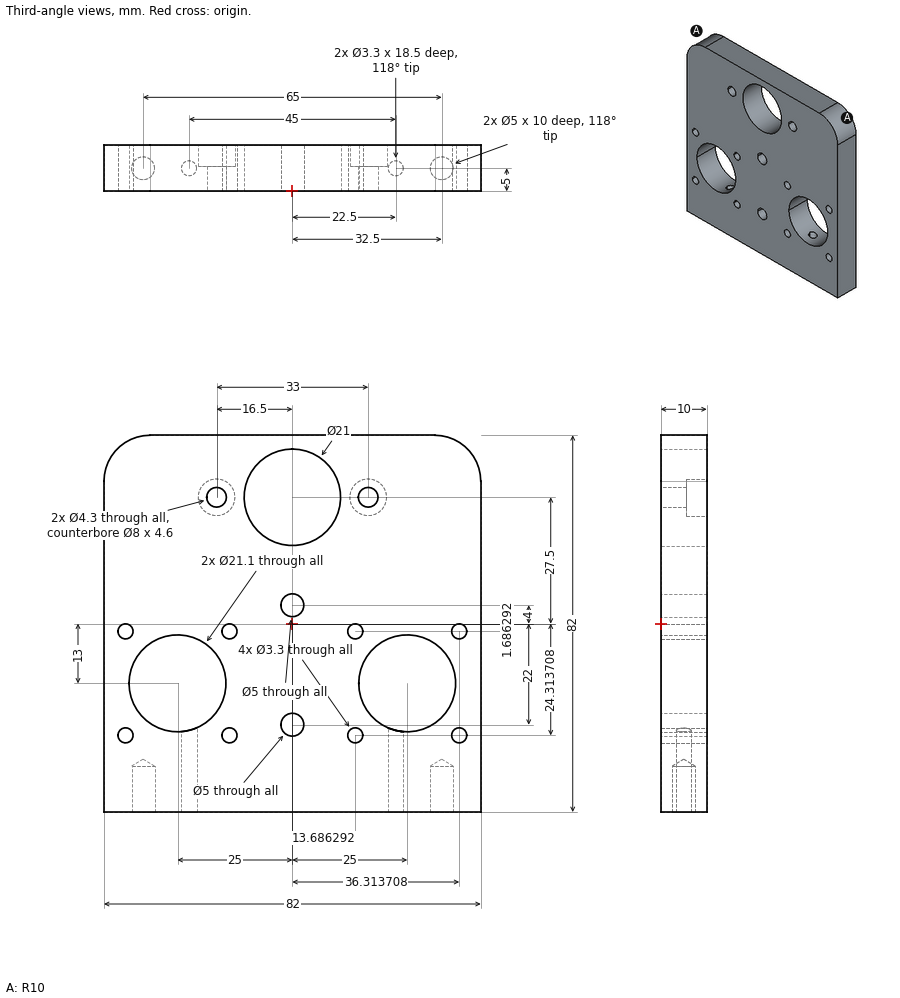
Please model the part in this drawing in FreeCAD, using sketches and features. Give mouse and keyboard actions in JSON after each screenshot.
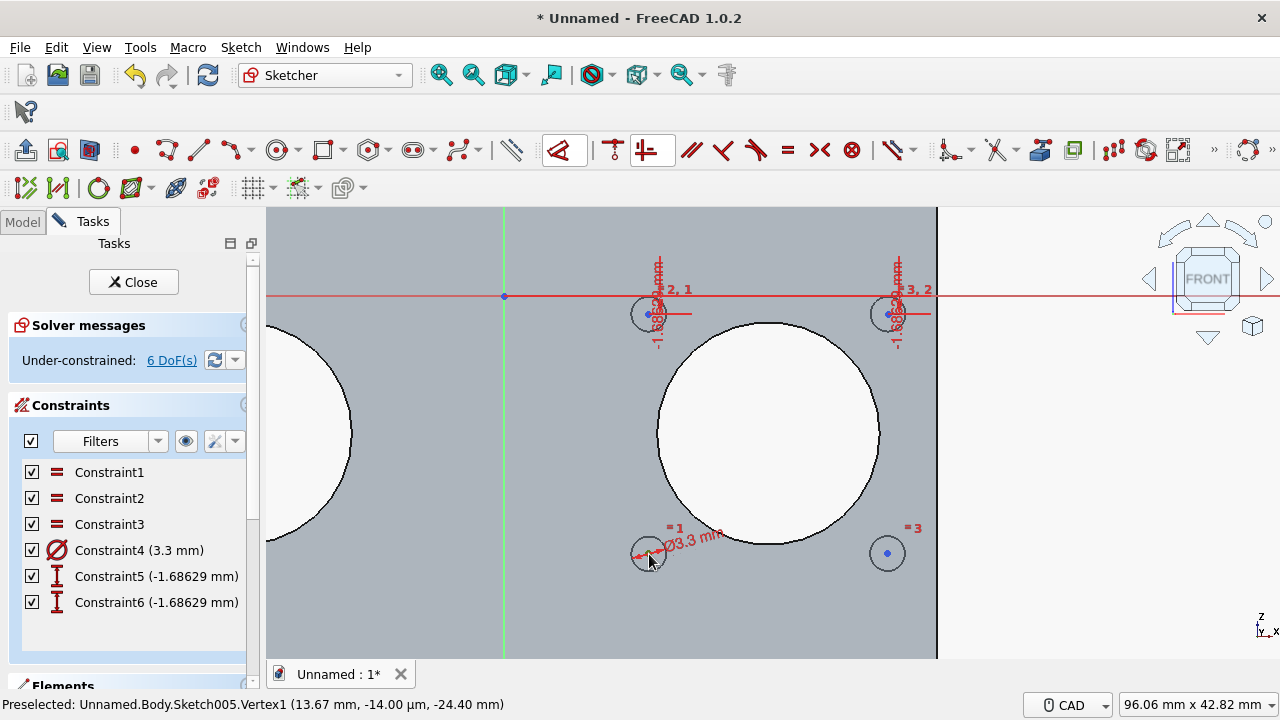
{"action": "key", "text": "l"}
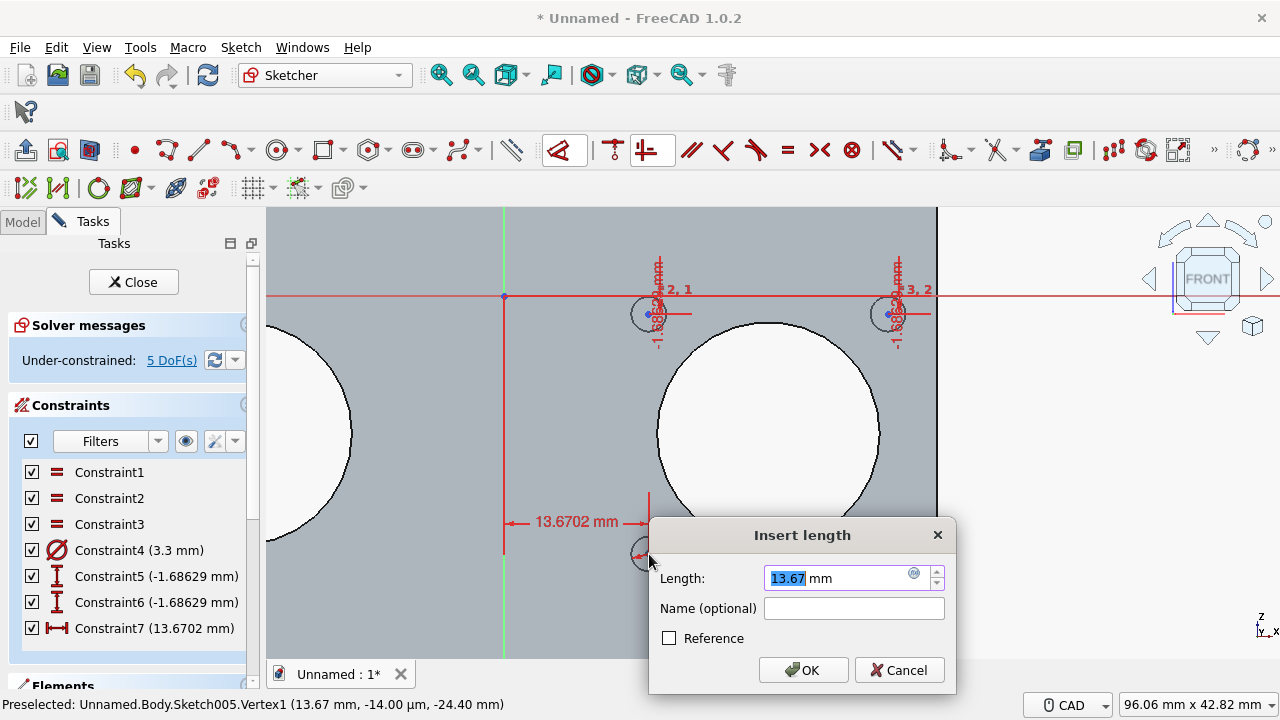
{"action": "type", "text": "13.686292"}
{"action": "key", "text": "Return"}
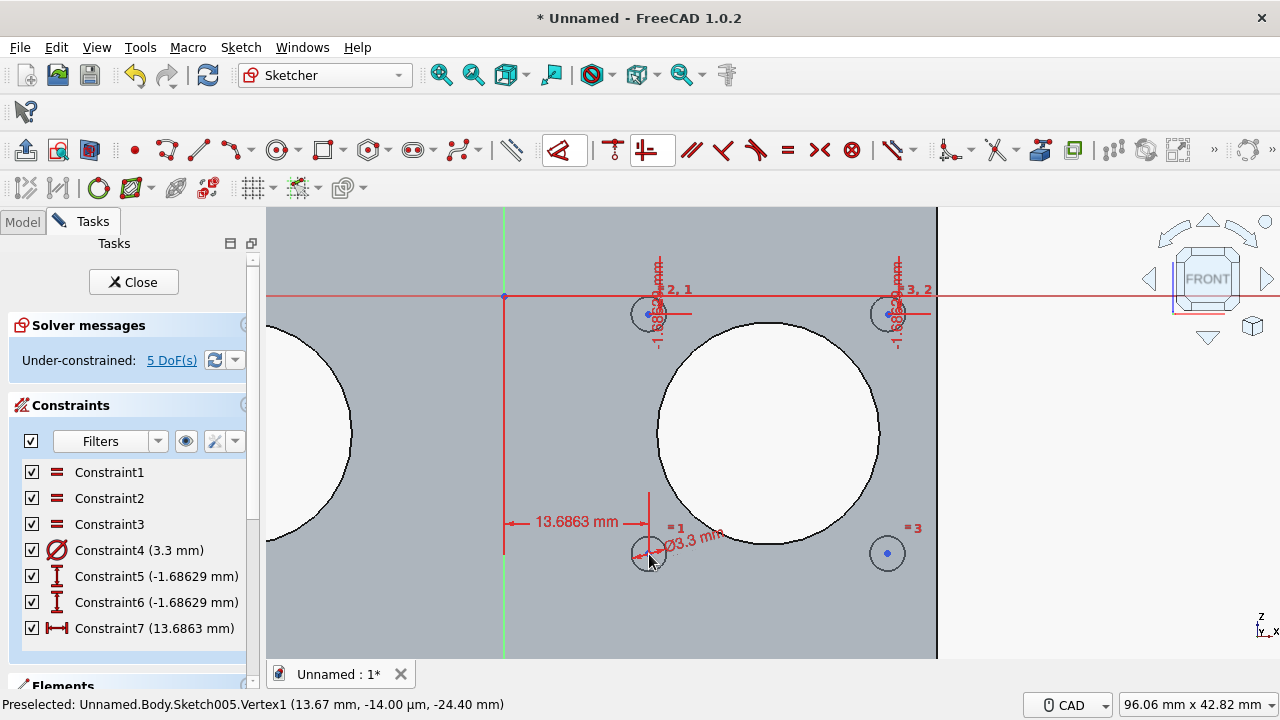
{"action": "left_click", "coordinate": [649, 554]}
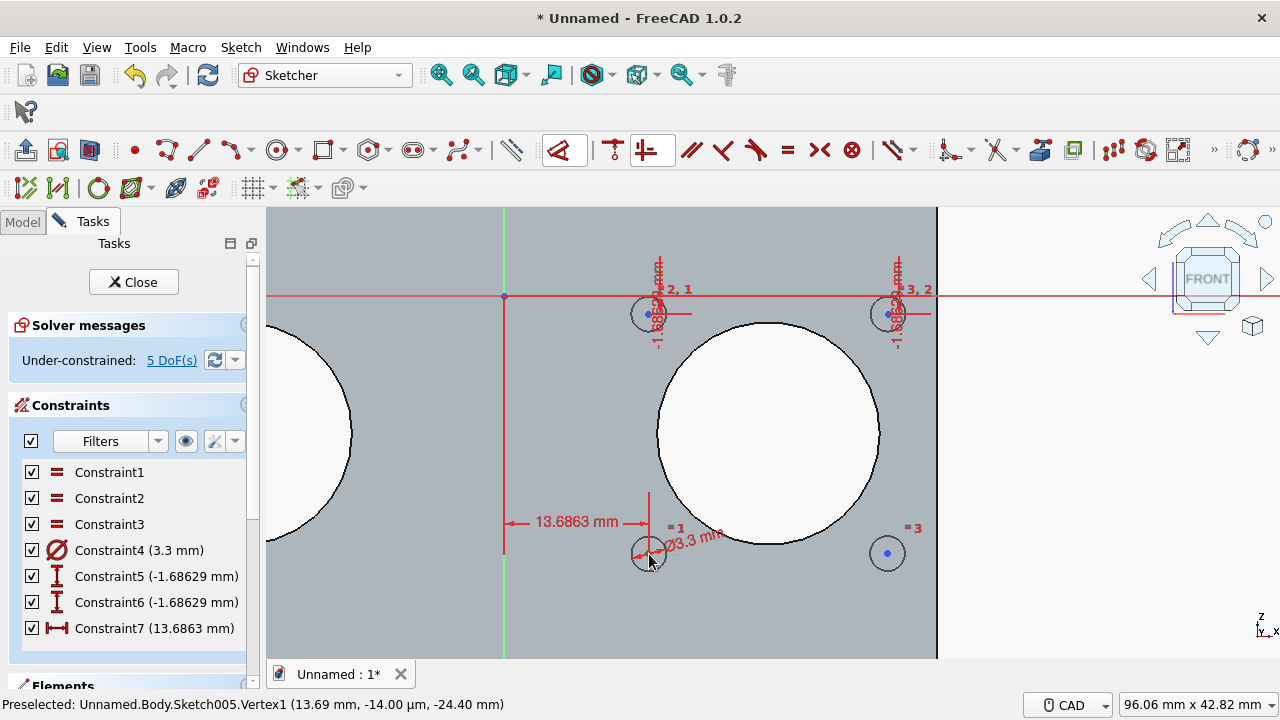
{"action": "key", "text": "i"}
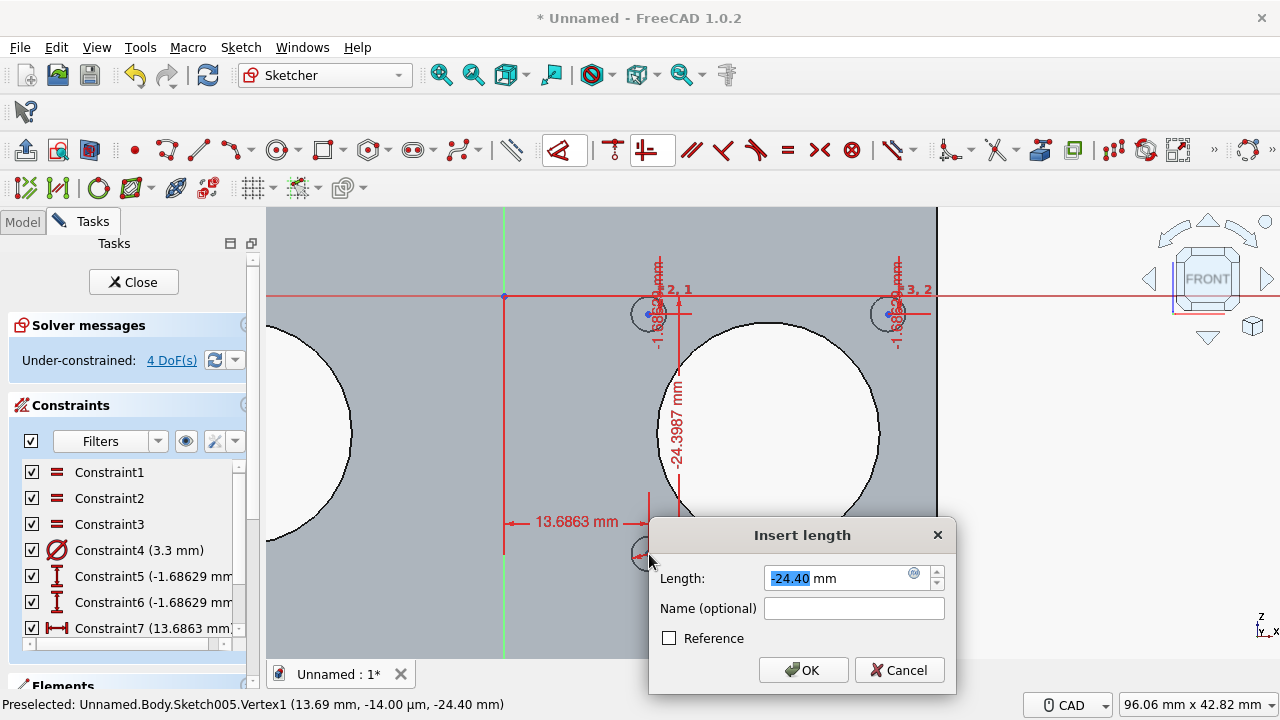
{"action": "type", "text": "-24.313708"}
{"action": "key", "text": "Return"}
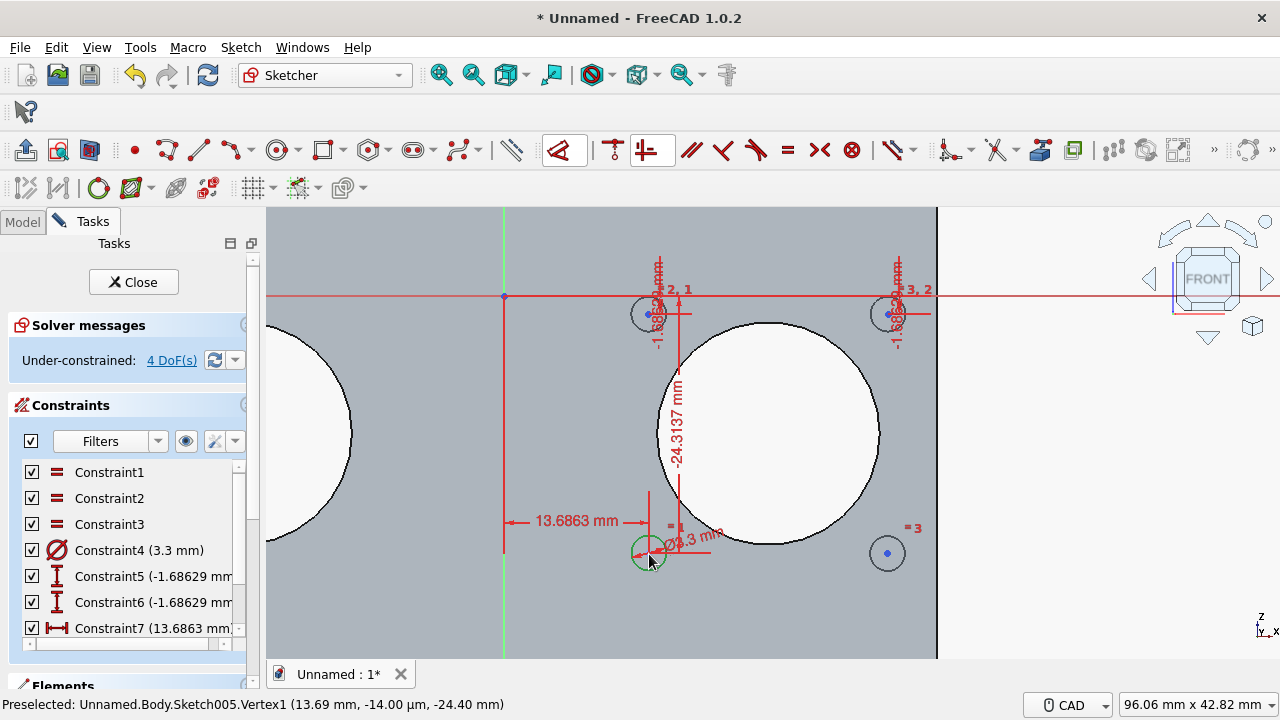
{"action": "left_click", "coordinate": [649, 314]}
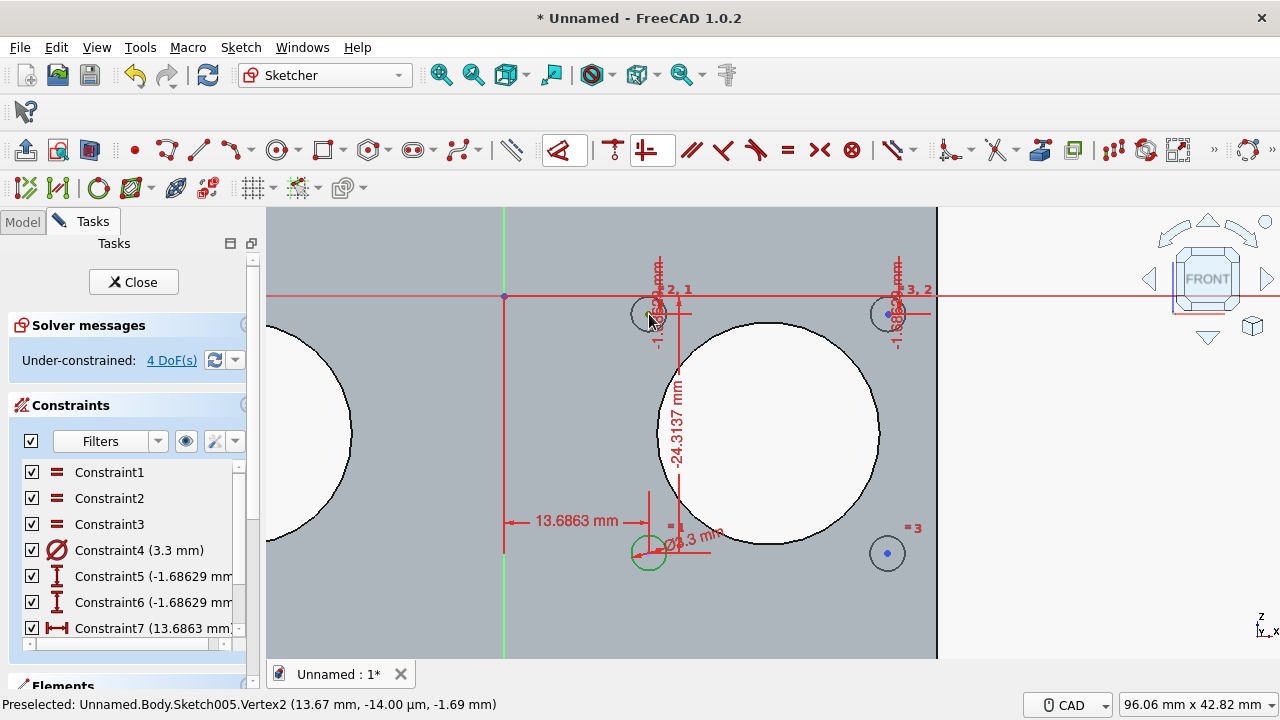
{"action": "key", "text": "l"}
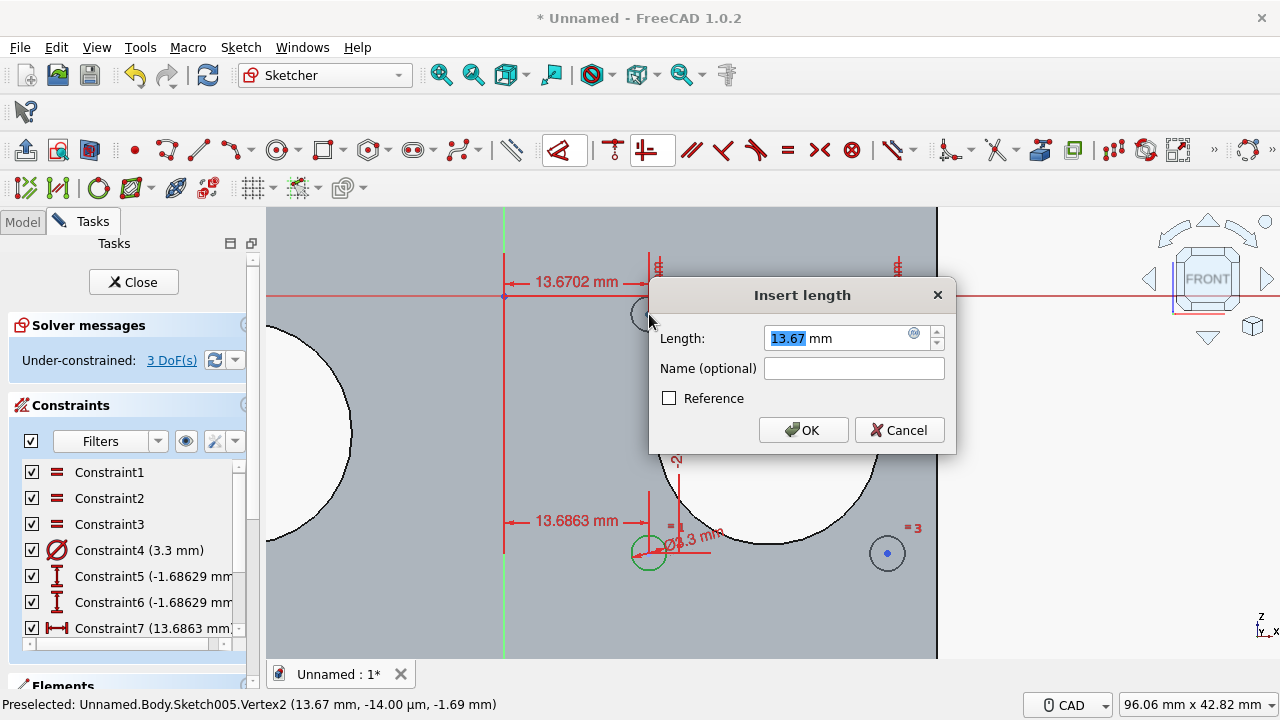
{"action": "type", "text": "13.686292"}
{"action": "key", "text": "Return"}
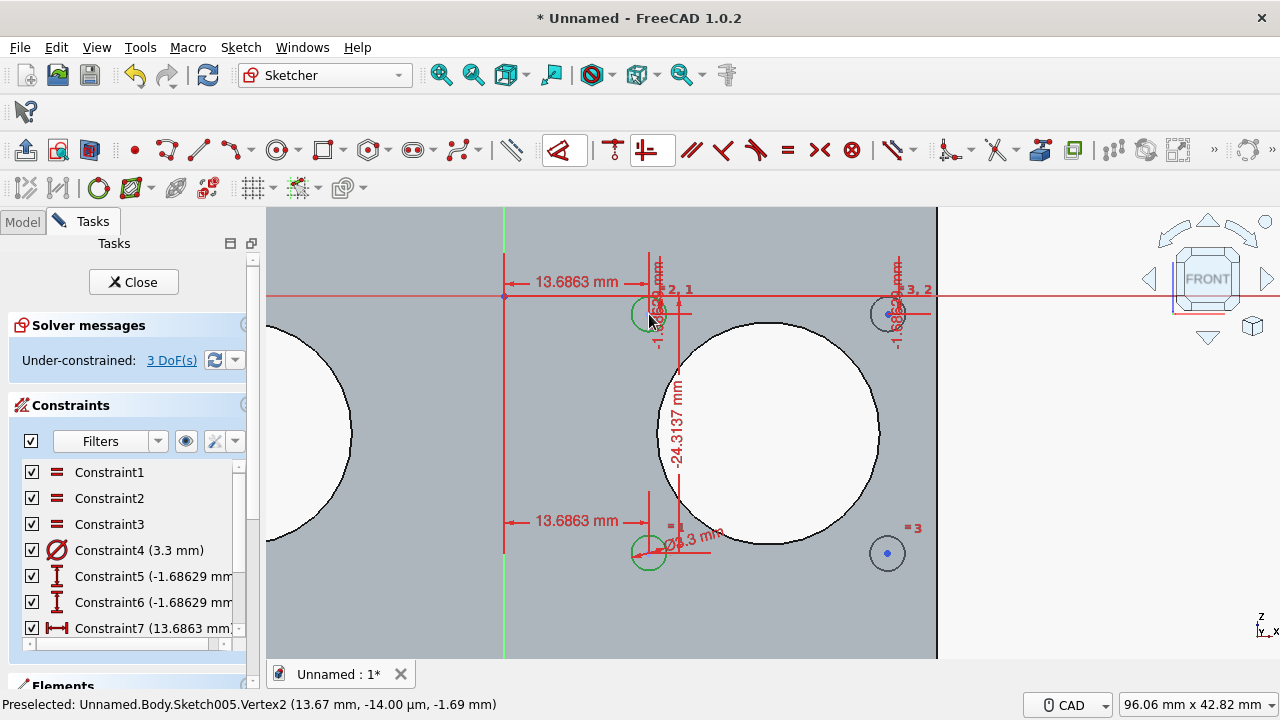
{"action": "left_click", "coordinate": [888, 314]}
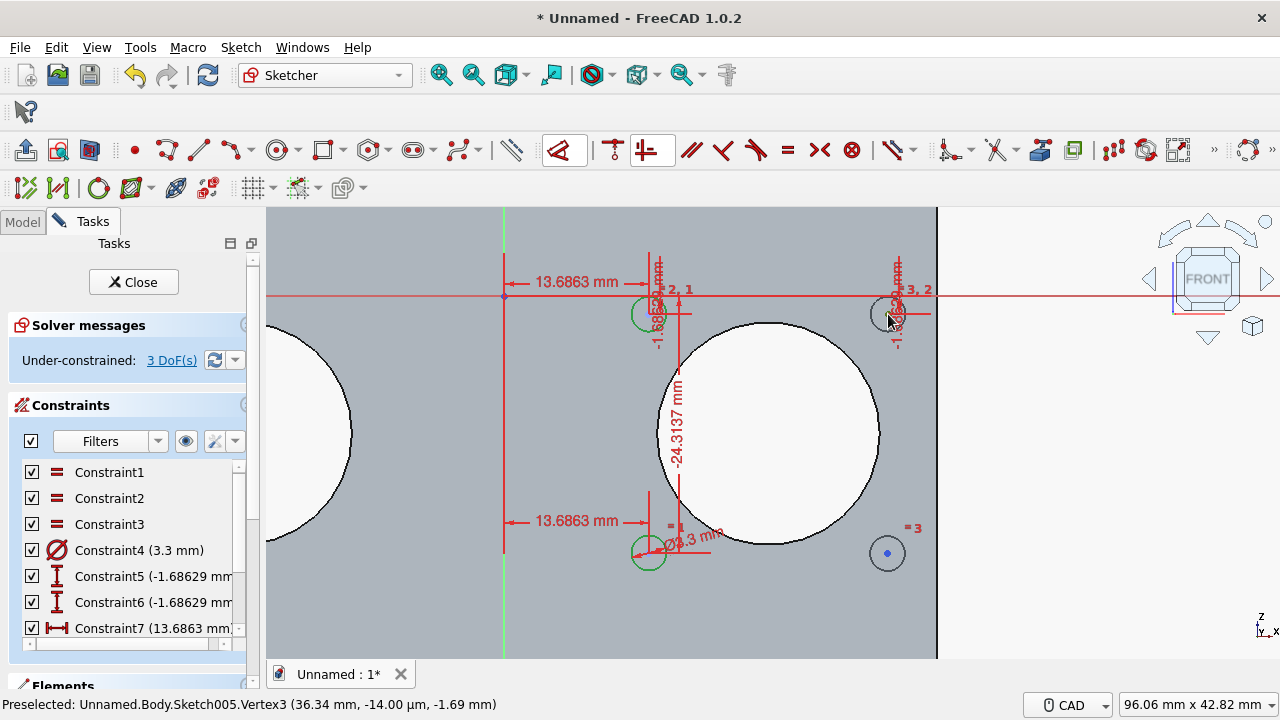
{"action": "key", "text": "l"}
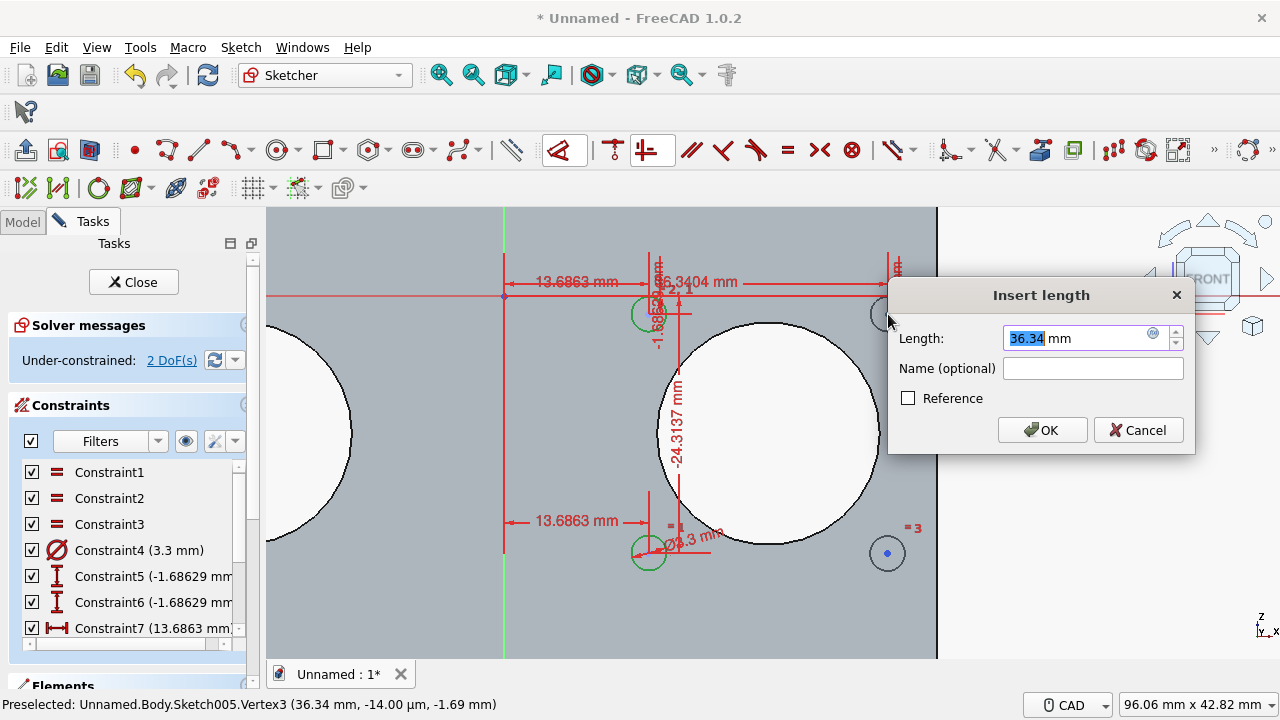
{"action": "type", "text": "36.313708"}
{"action": "key", "text": "Return"}